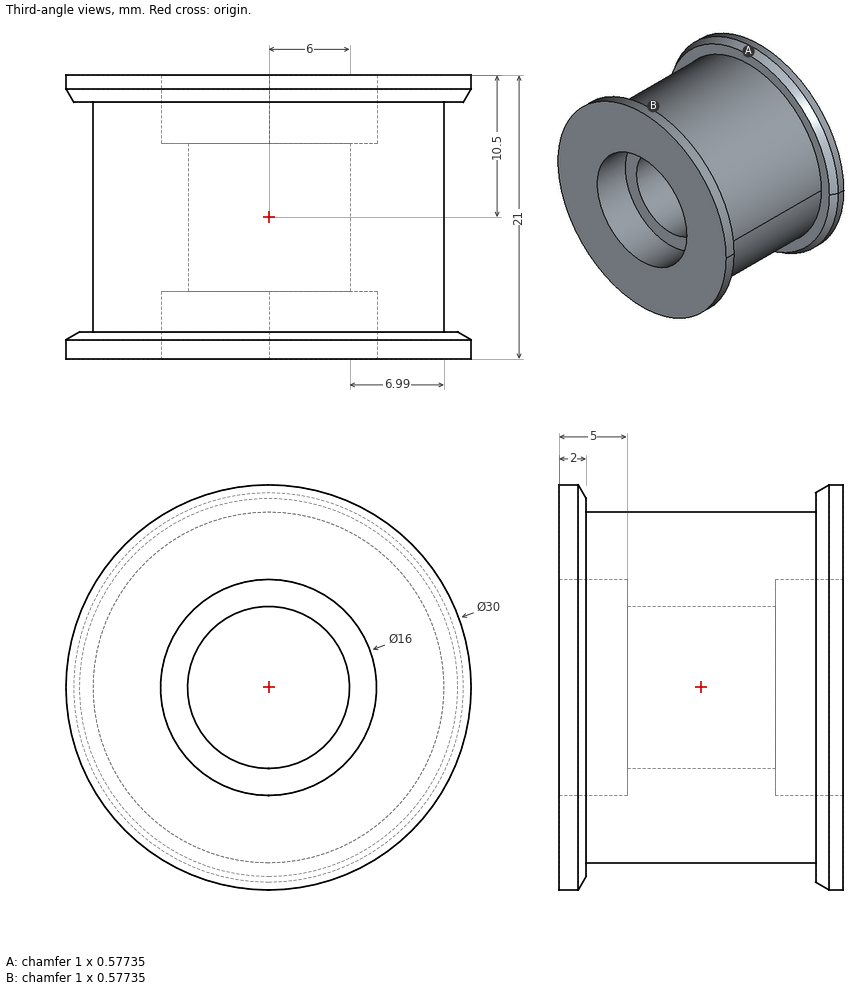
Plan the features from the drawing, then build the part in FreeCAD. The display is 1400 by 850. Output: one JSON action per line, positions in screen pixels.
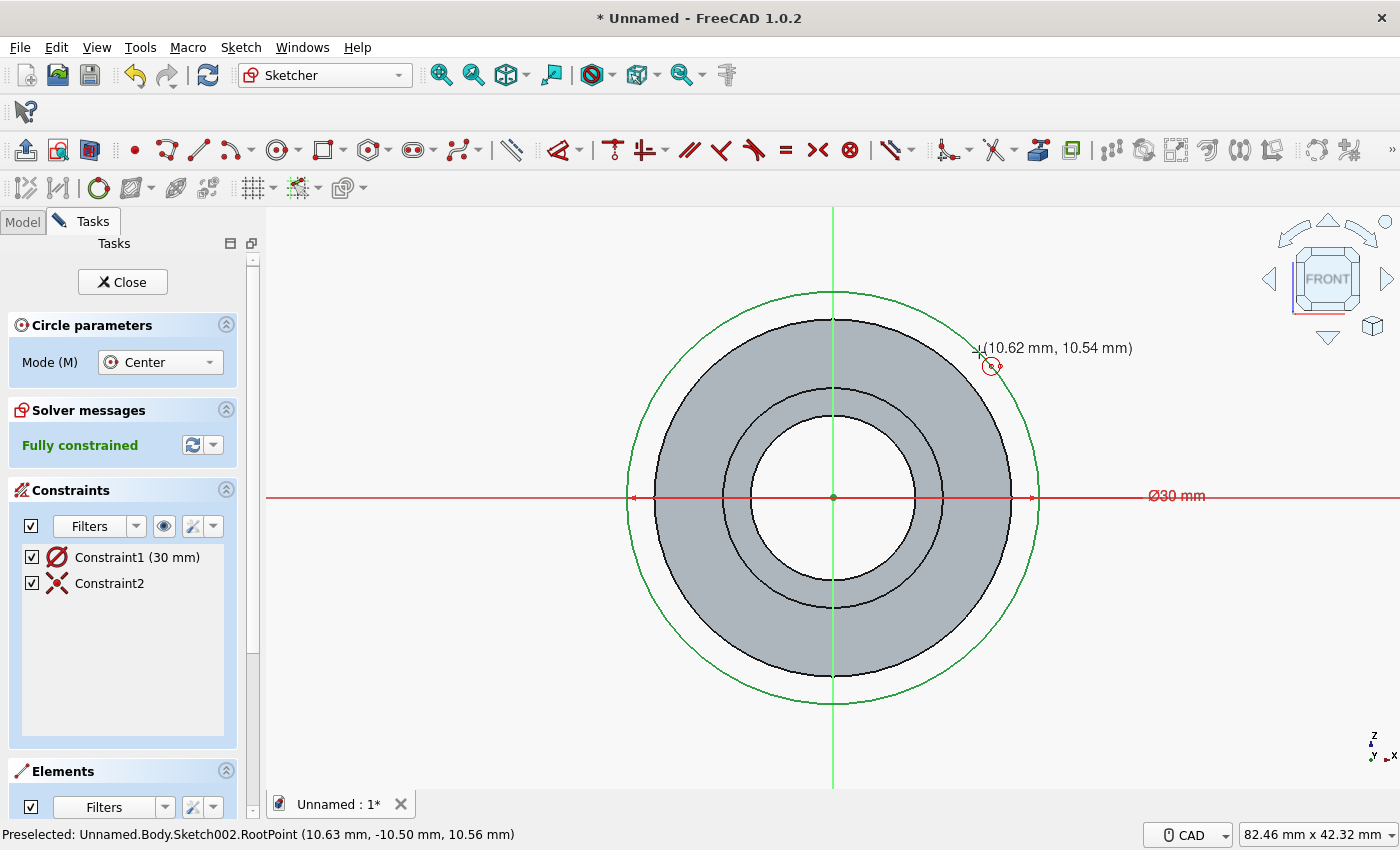
{"action": "left_click", "coordinate": [833, 498]}
{"action": "mouse_move", "coordinate": [911, 420]}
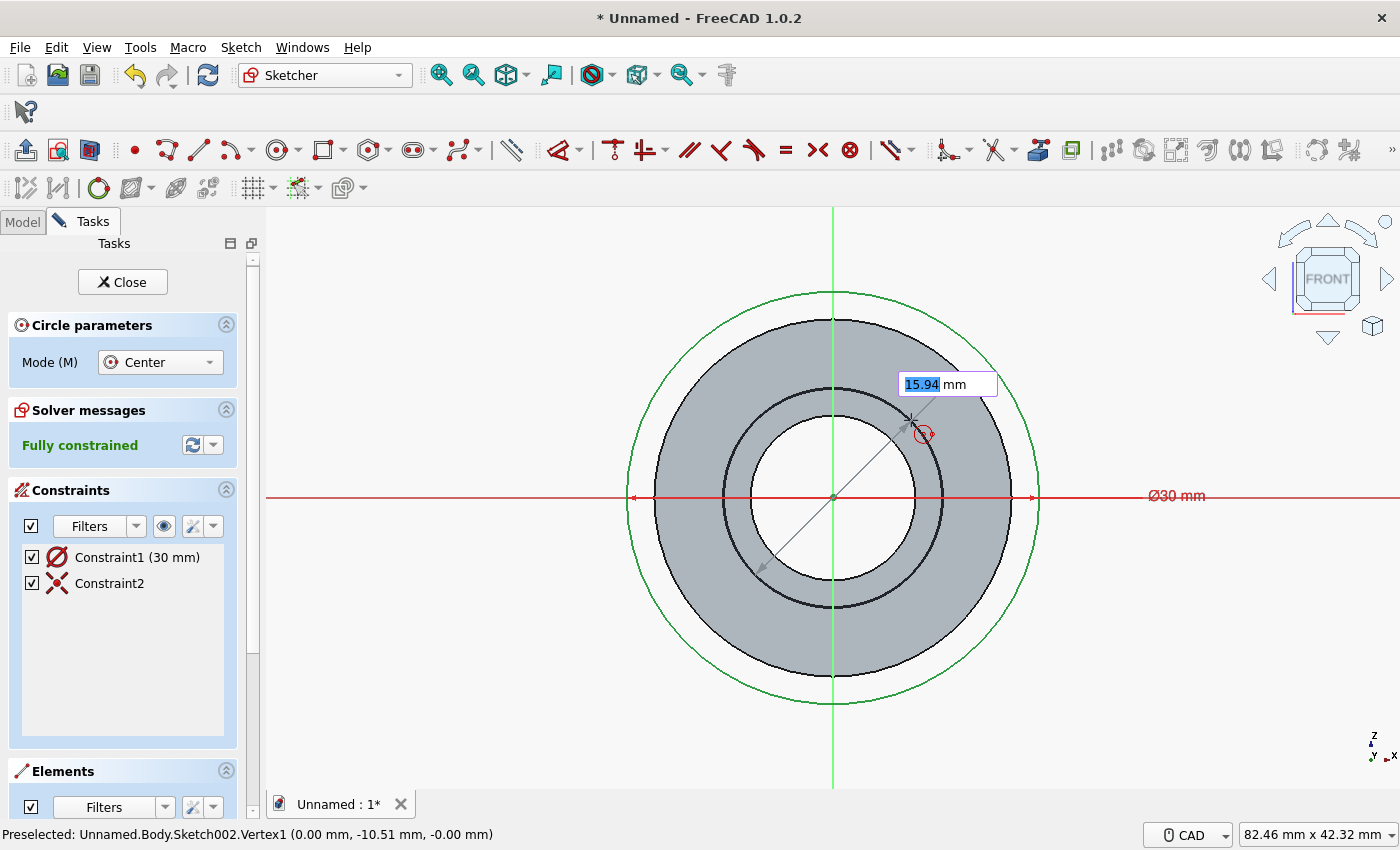
{"action": "type", "text": "16"}
{"action": "key", "text": "Return"}
{"action": "key", "text": "Escape"}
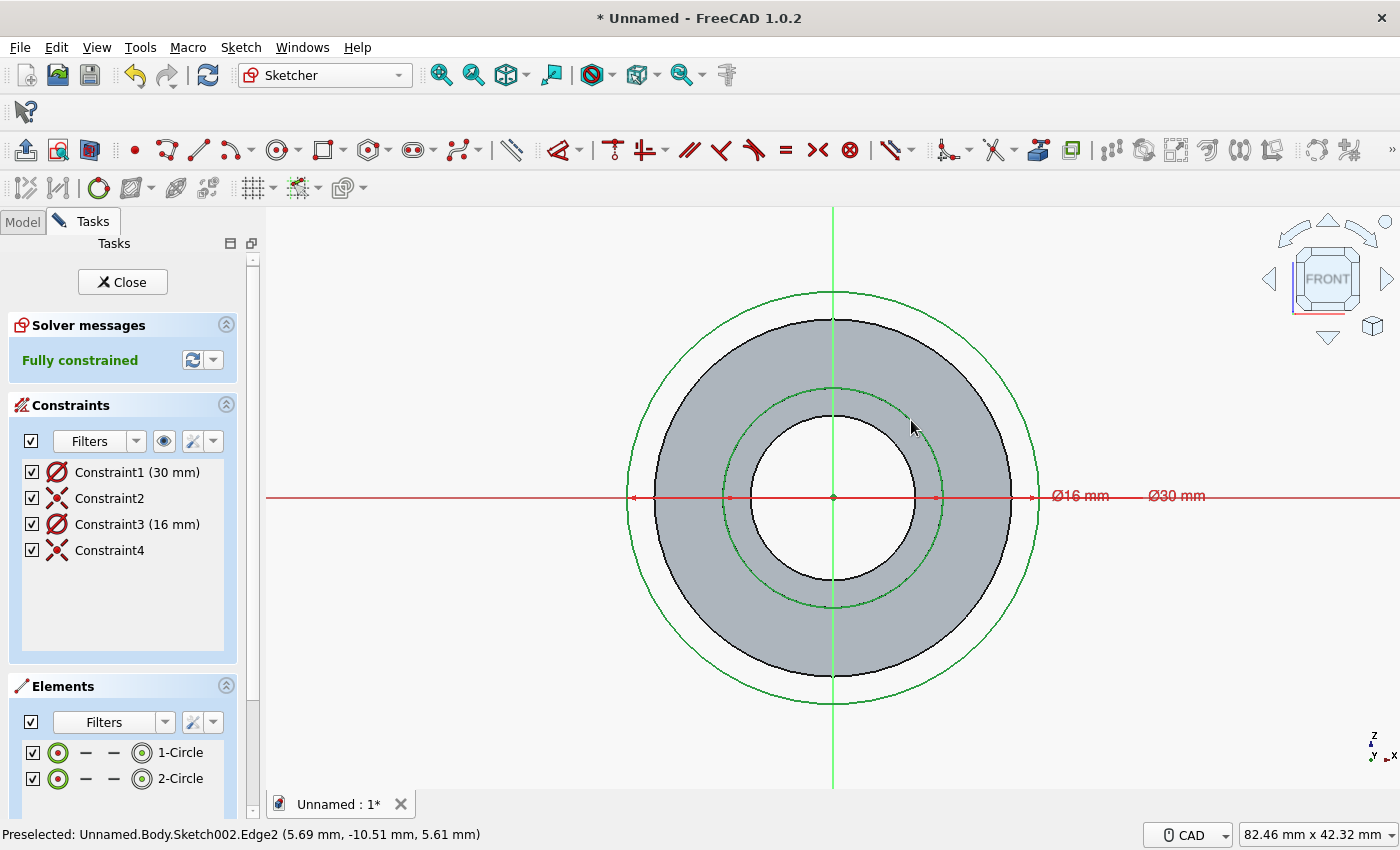
{"action": "left_click", "coordinate": [123, 282]}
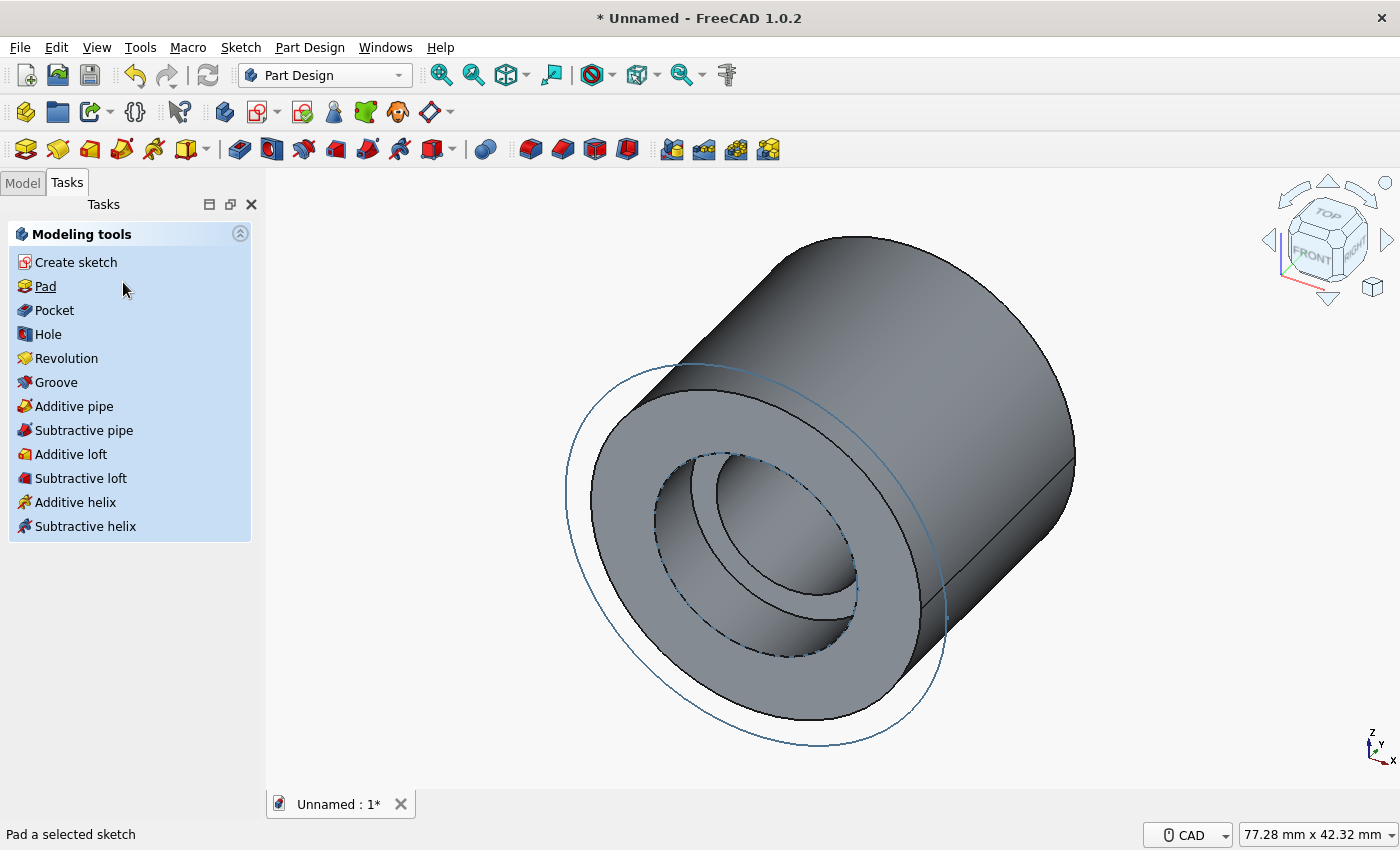
{"action": "left_click", "coordinate": [26, 150]}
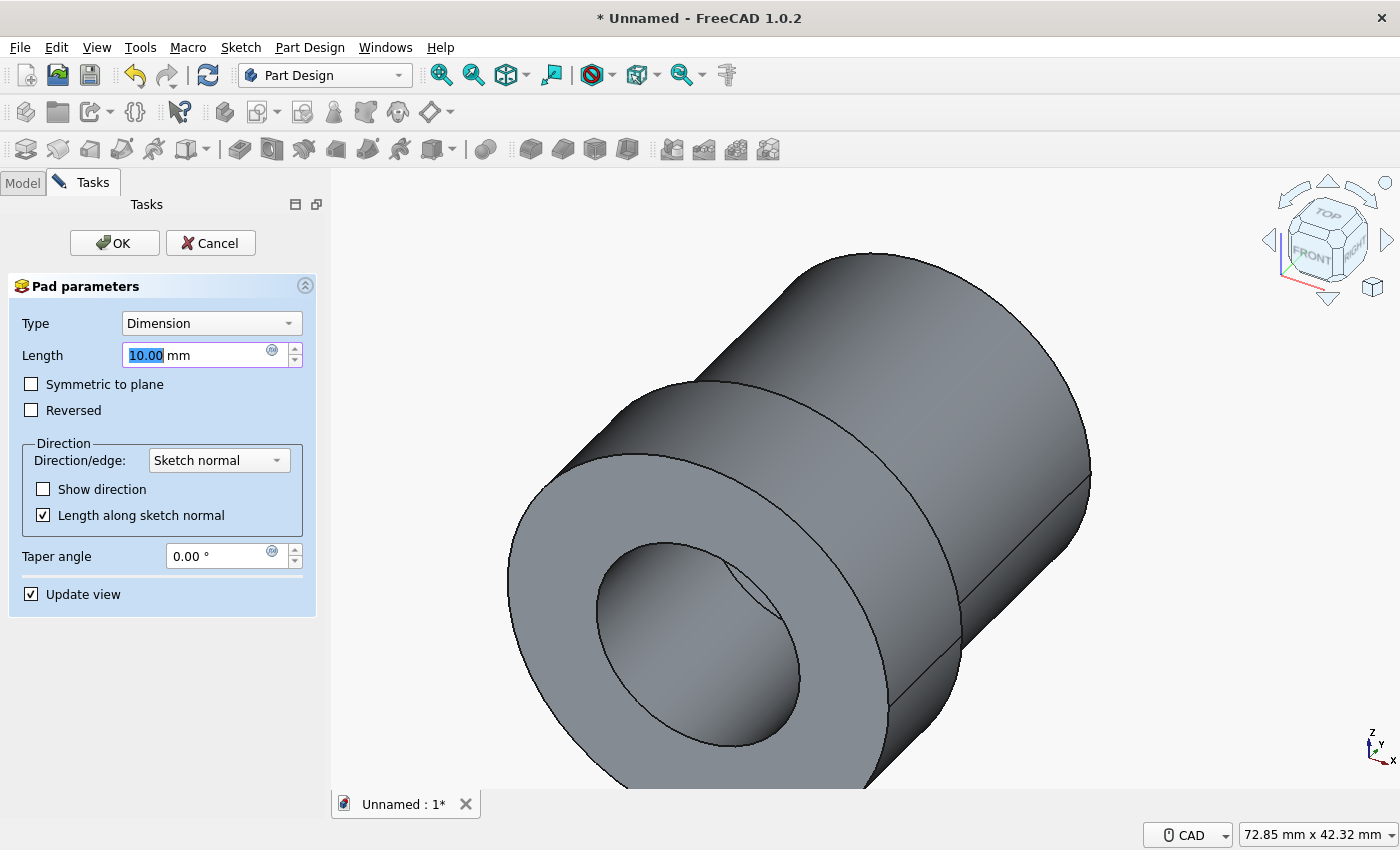
{"action": "type", "text": "2"}
{"action": "key", "text": "Tab"}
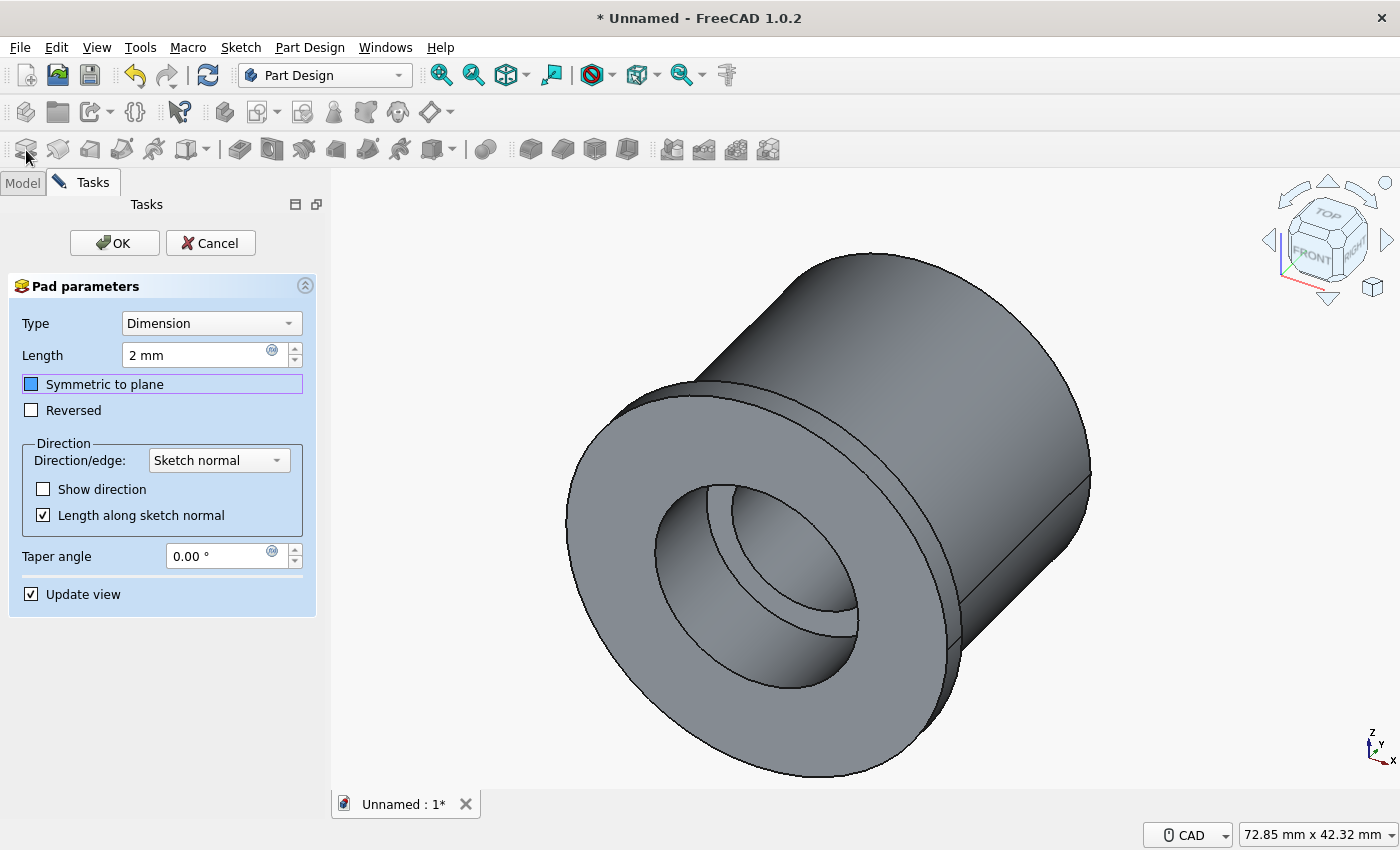
{"action": "left_click", "coordinate": [30, 410]}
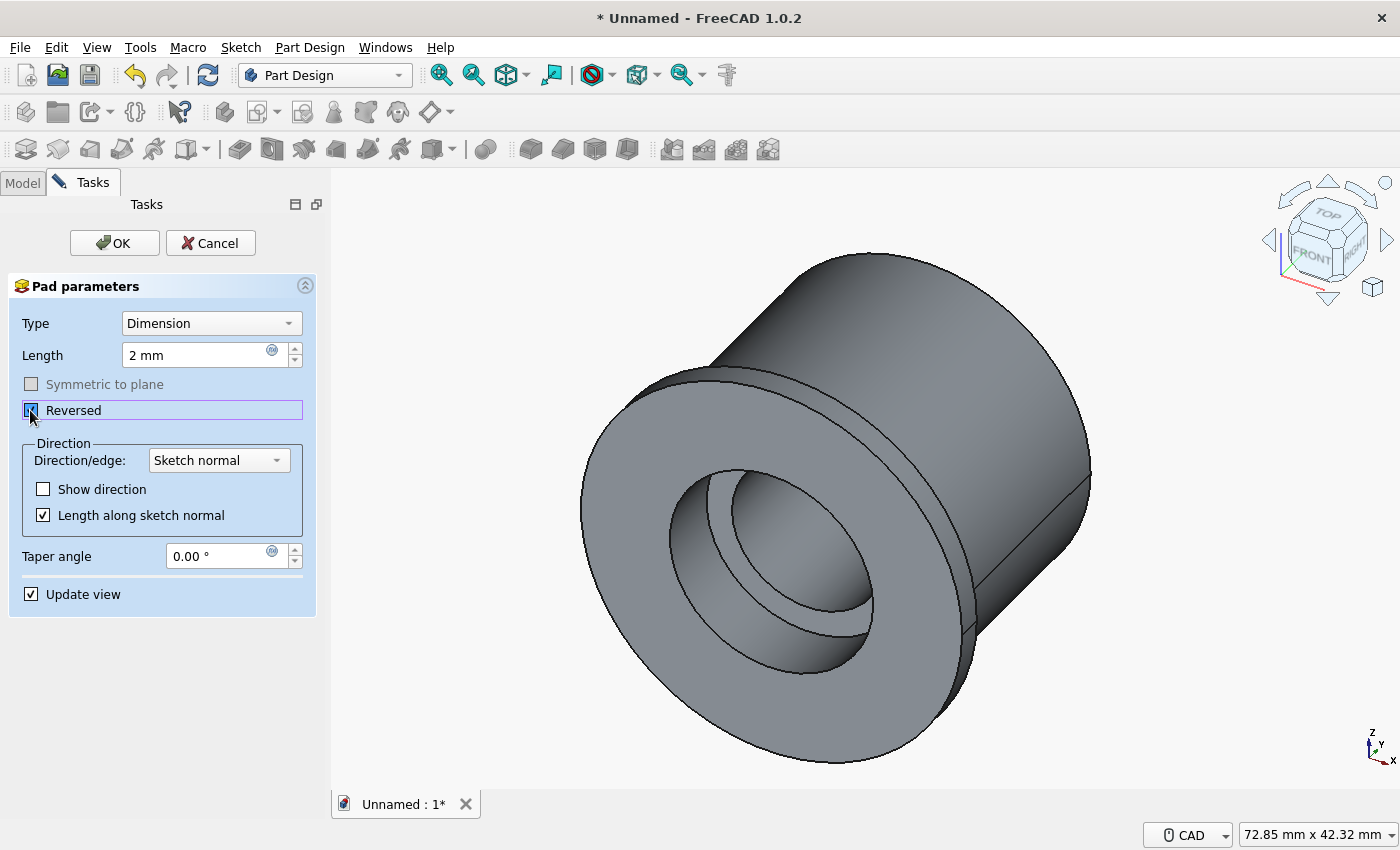
{"action": "left_click", "coordinate": [115, 243]}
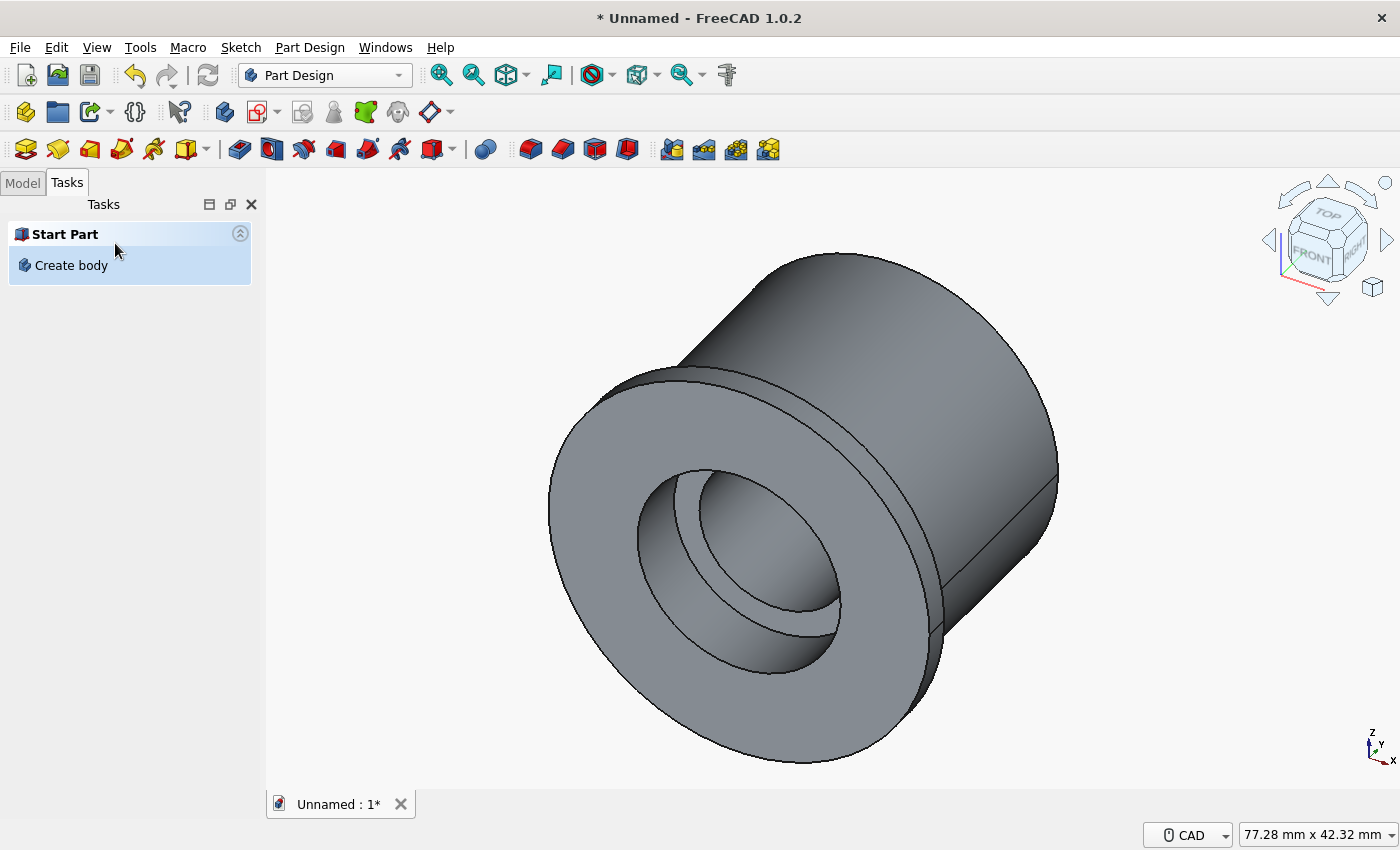
{"action": "left_click", "coordinate": [442, 76]}